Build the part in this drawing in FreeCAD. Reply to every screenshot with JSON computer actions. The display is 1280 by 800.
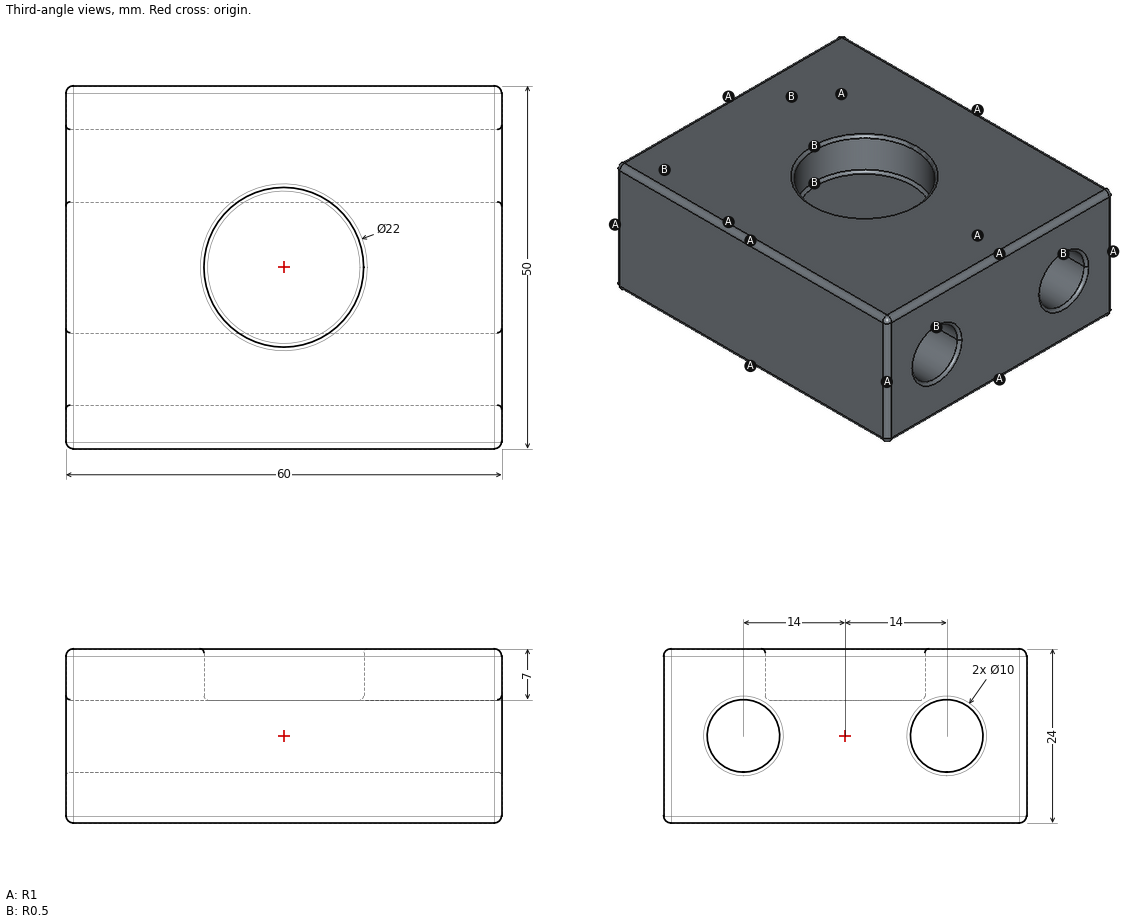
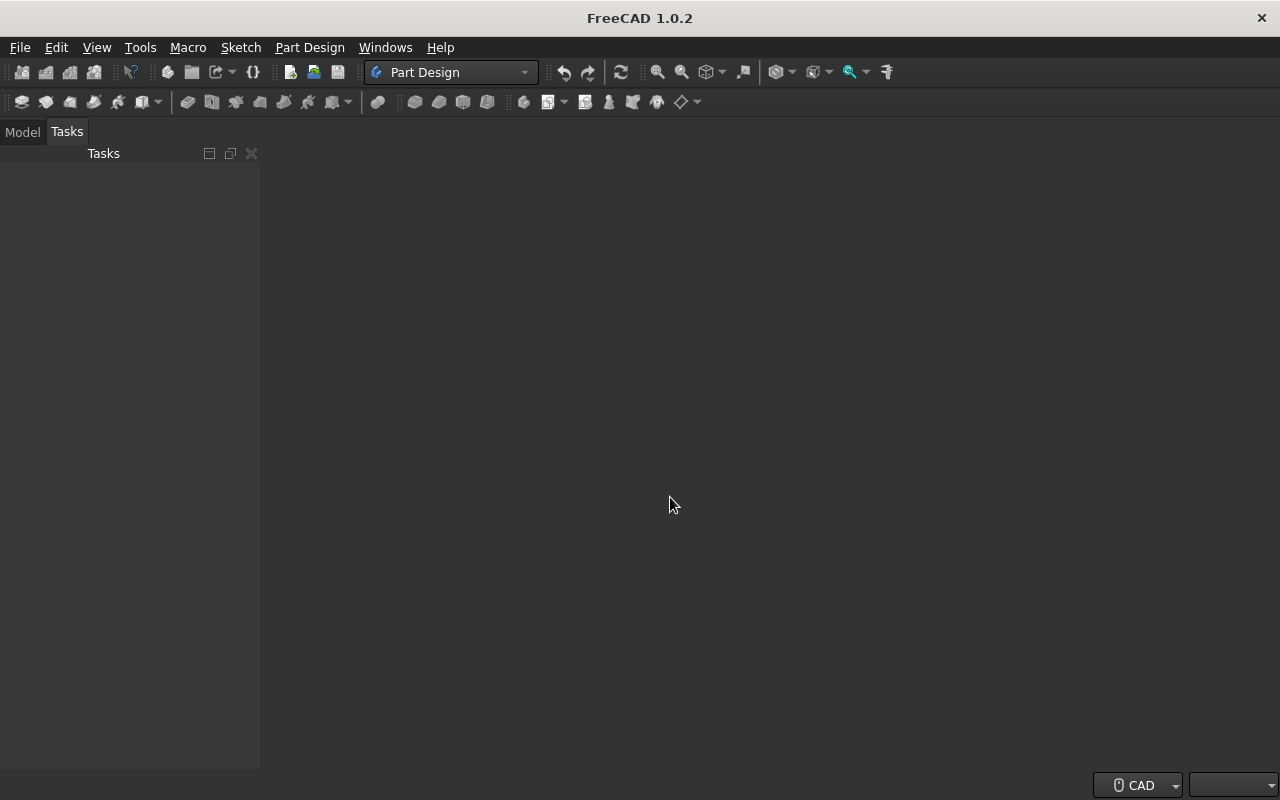
{"action": "left_click", "coordinate": [290, 72]}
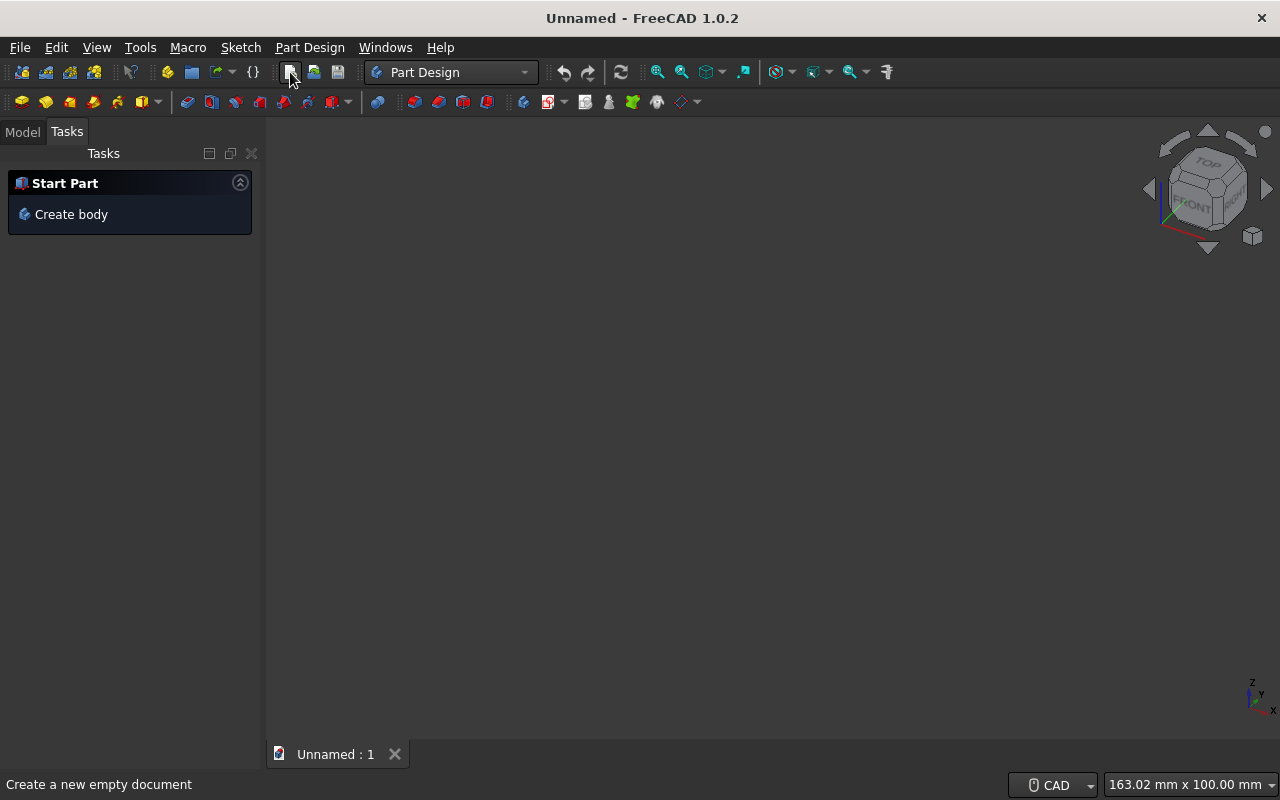
{"action": "left_click", "coordinate": [548, 102]}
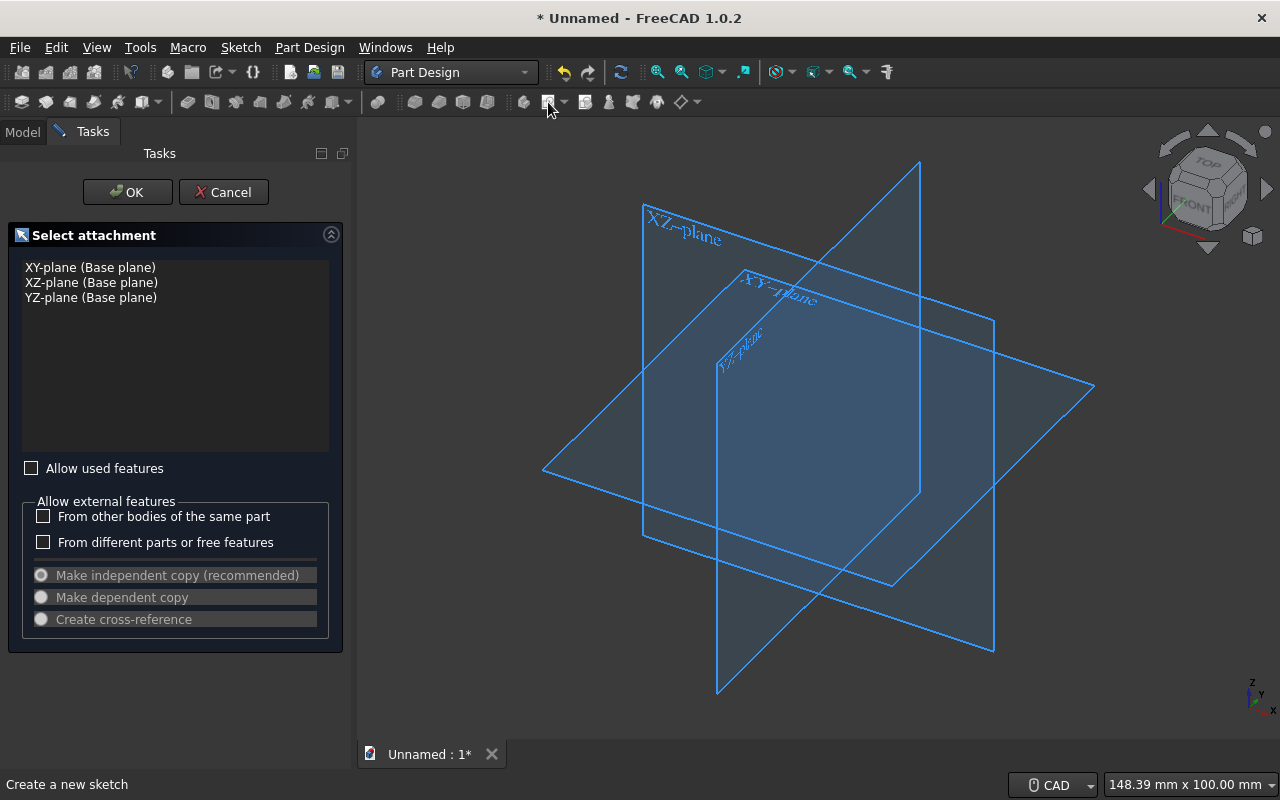
{"action": "left_click", "coordinate": [82, 268]}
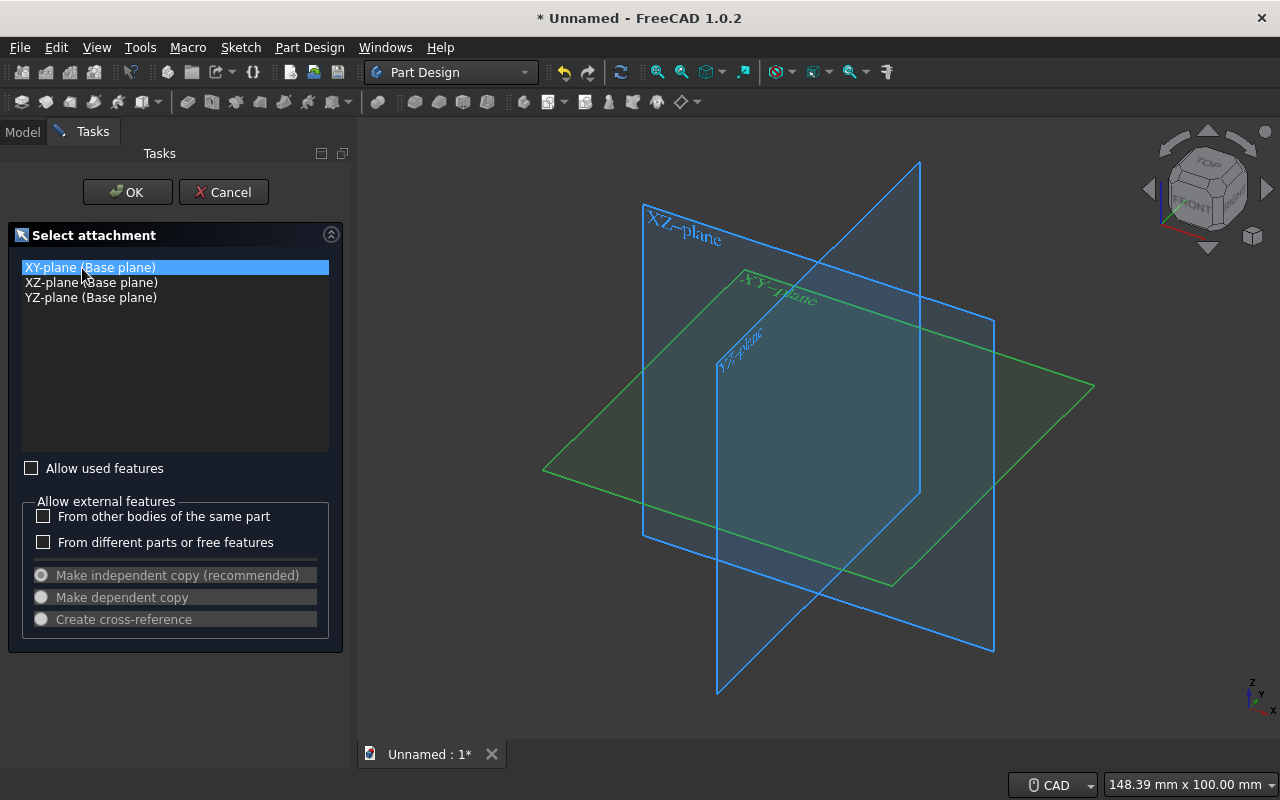
{"action": "left_click", "coordinate": [128, 192]}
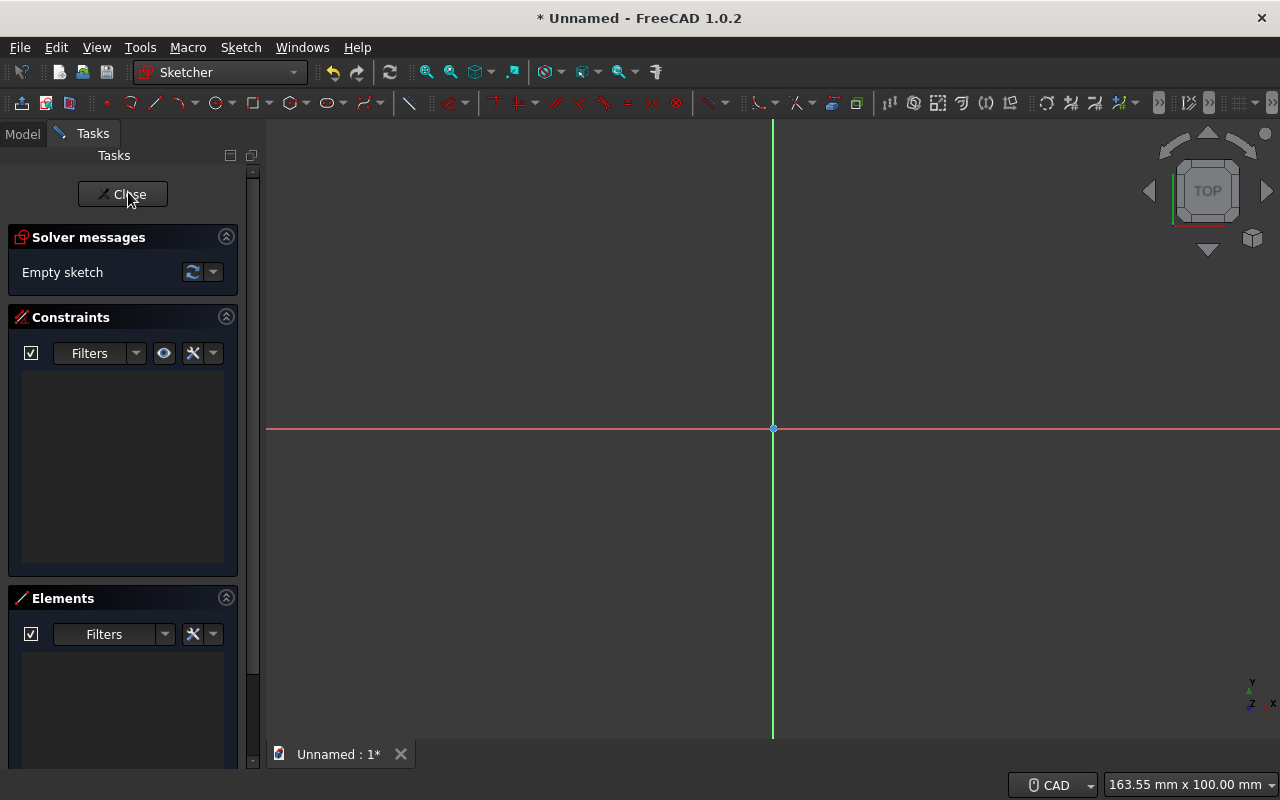
{"action": "left_click", "coordinate": [272, 104]}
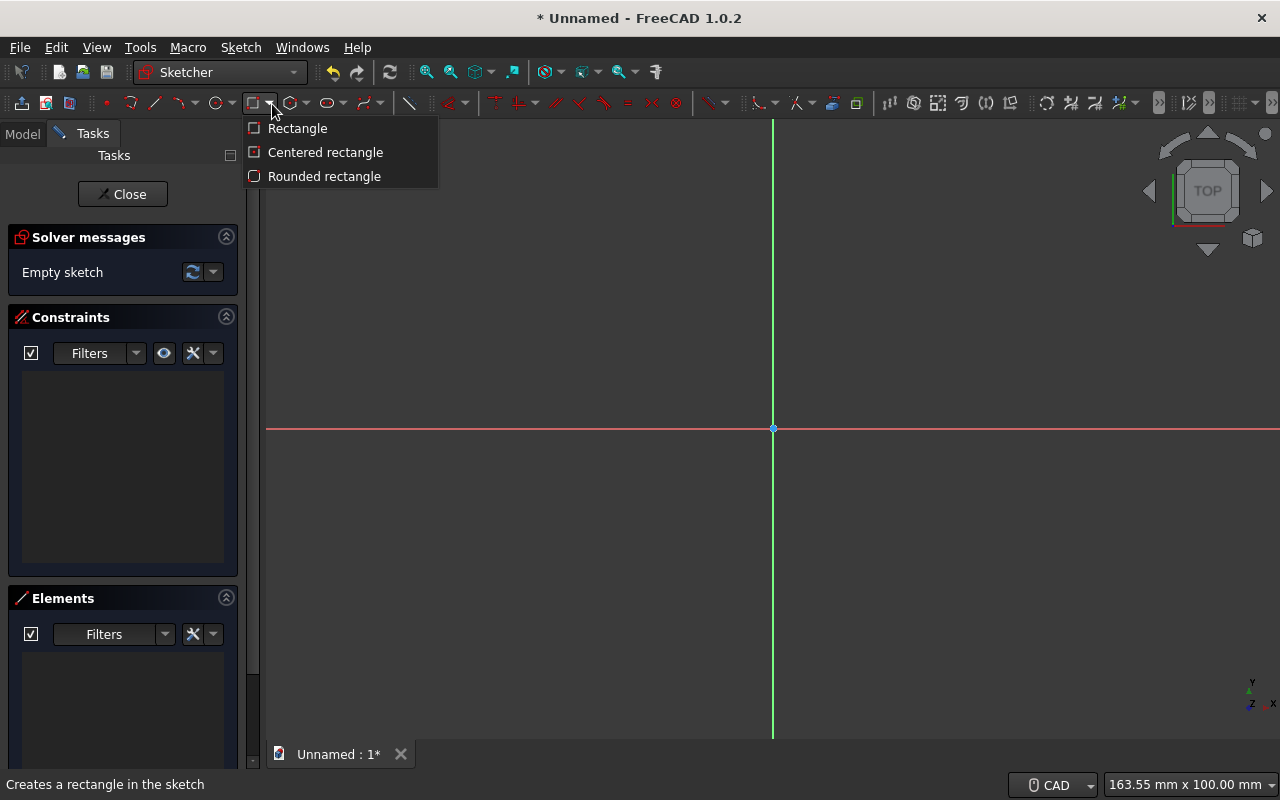
{"action": "left_click", "coordinate": [340, 152]}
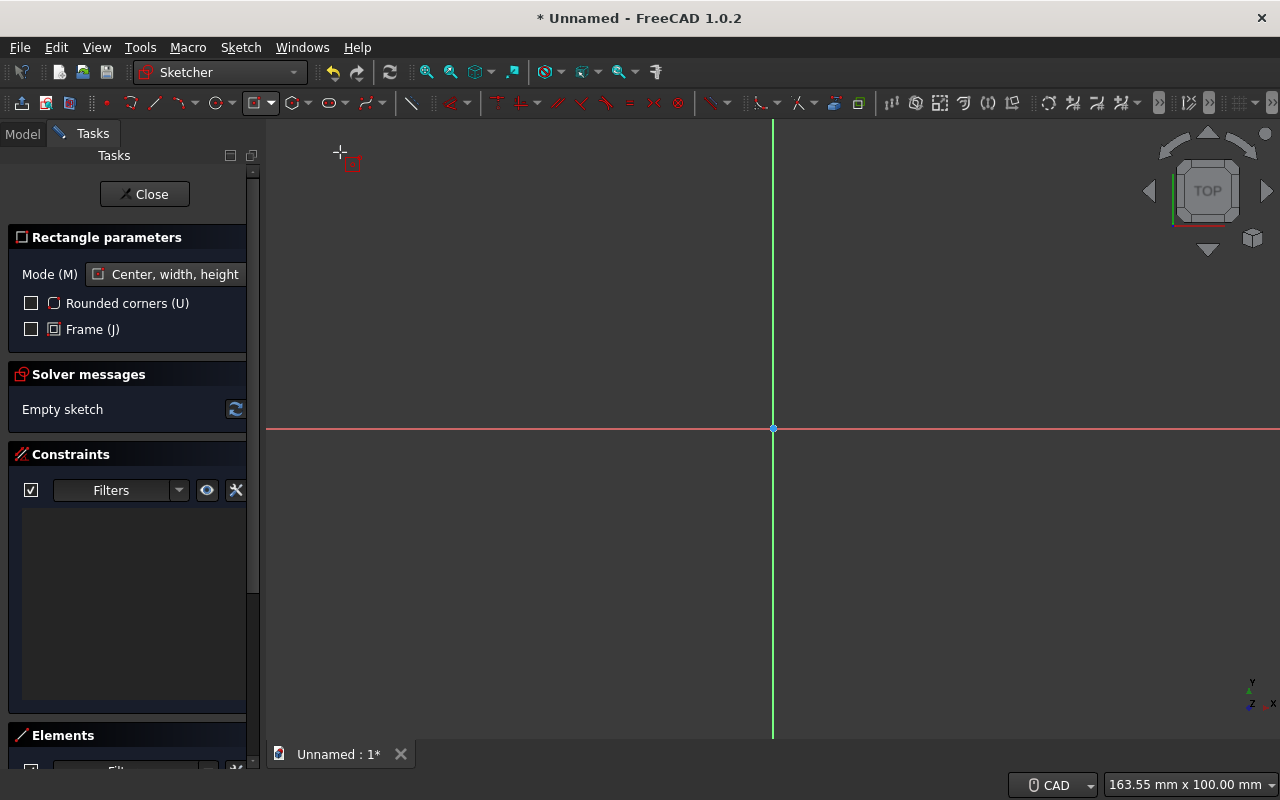
{"action": "left_click", "coordinate": [773, 429]}
{"action": "mouse_move", "coordinate": [959, 274]}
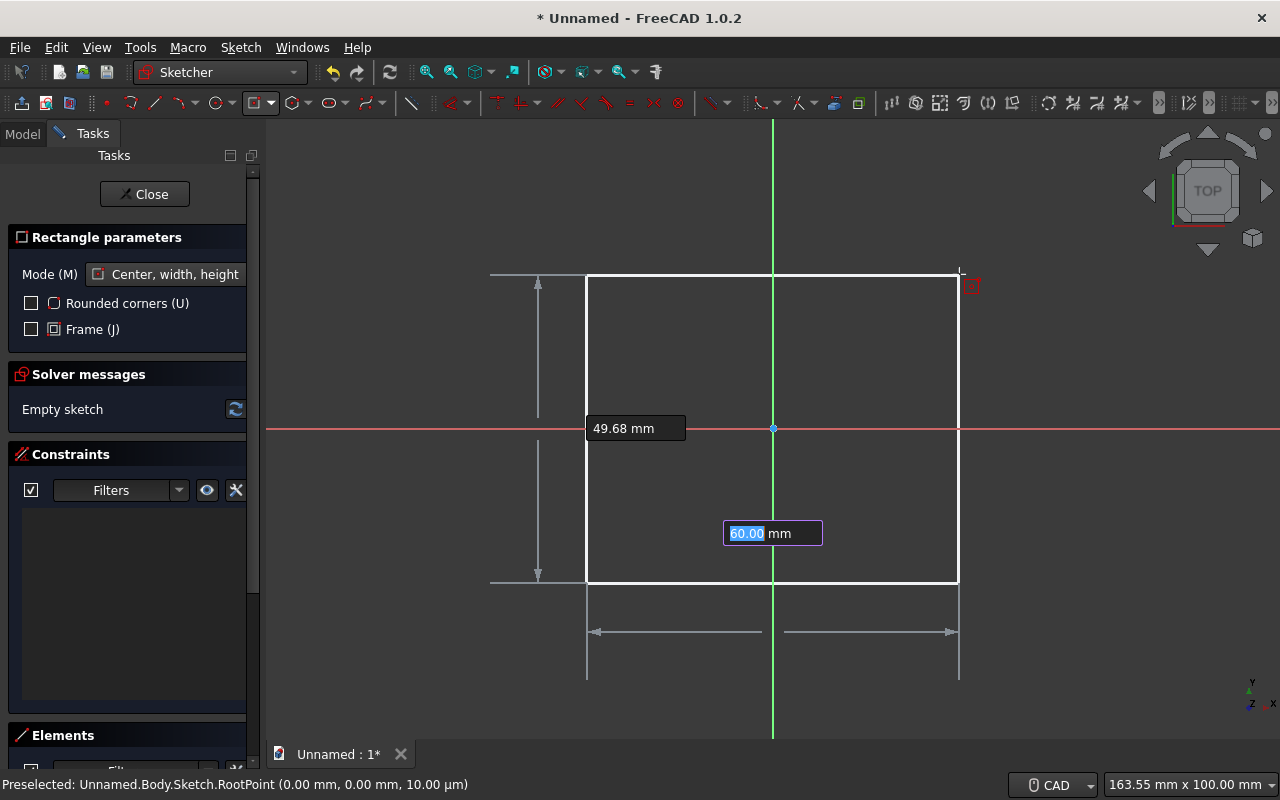
{"action": "type", "text": "60"}
{"action": "key", "text": "Tab"}
{"action": "type", "text": "50"}
{"action": "key", "text": "Return"}
{"action": "key", "text": "Escape"}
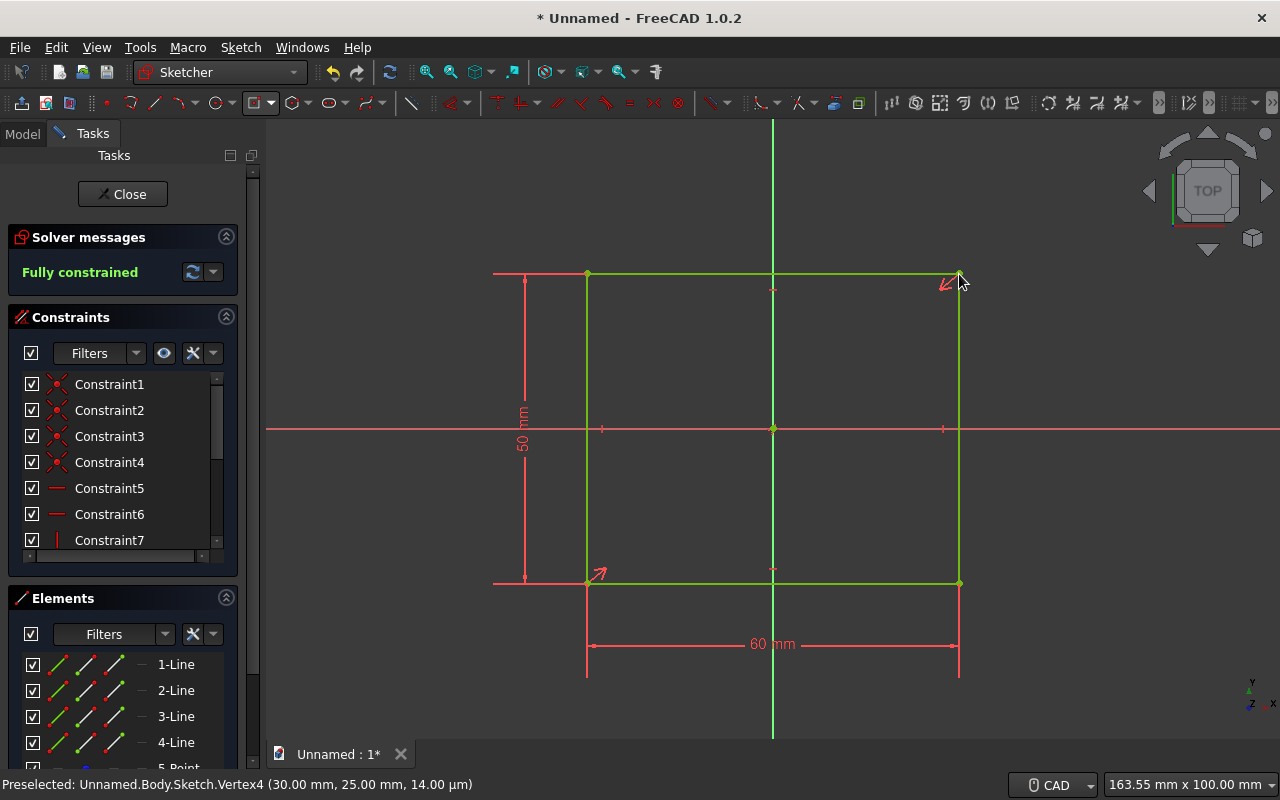
{"action": "left_click", "coordinate": [123, 194]}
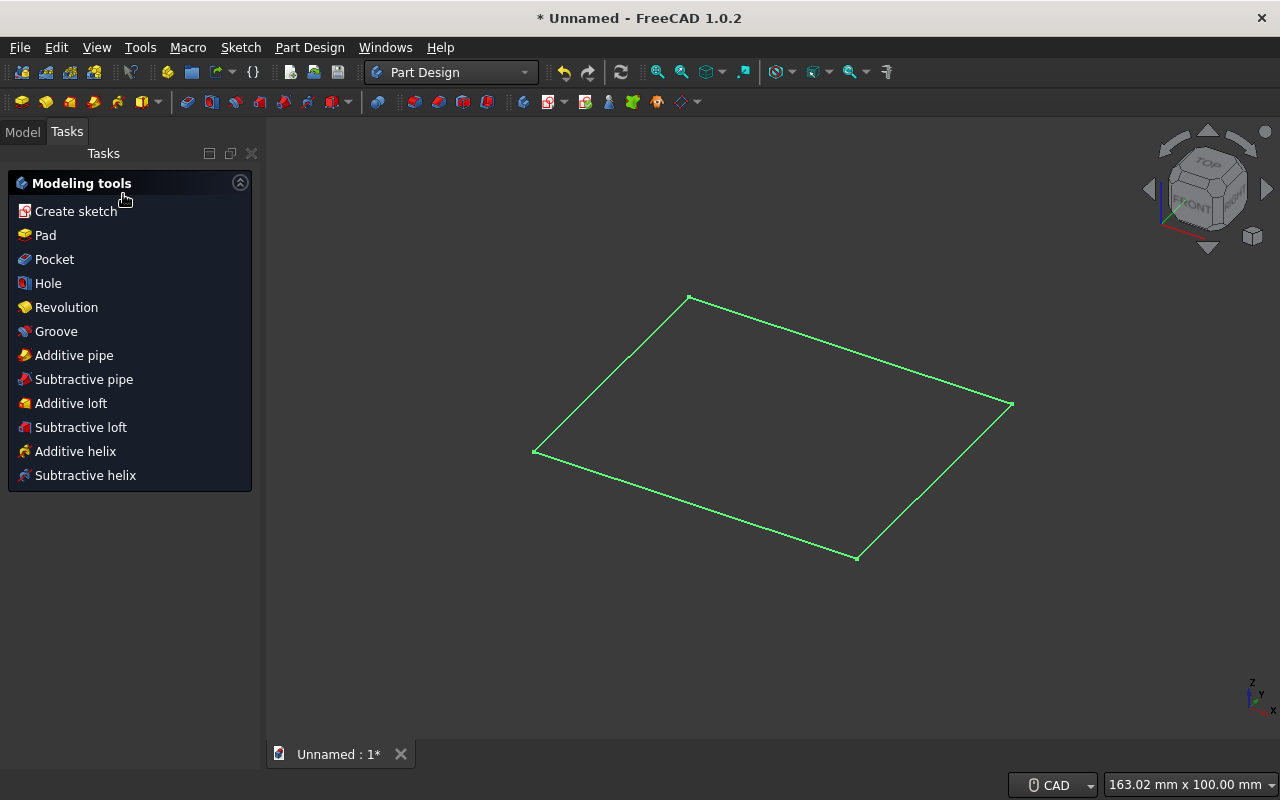
{"action": "left_click", "coordinate": [22, 102]}